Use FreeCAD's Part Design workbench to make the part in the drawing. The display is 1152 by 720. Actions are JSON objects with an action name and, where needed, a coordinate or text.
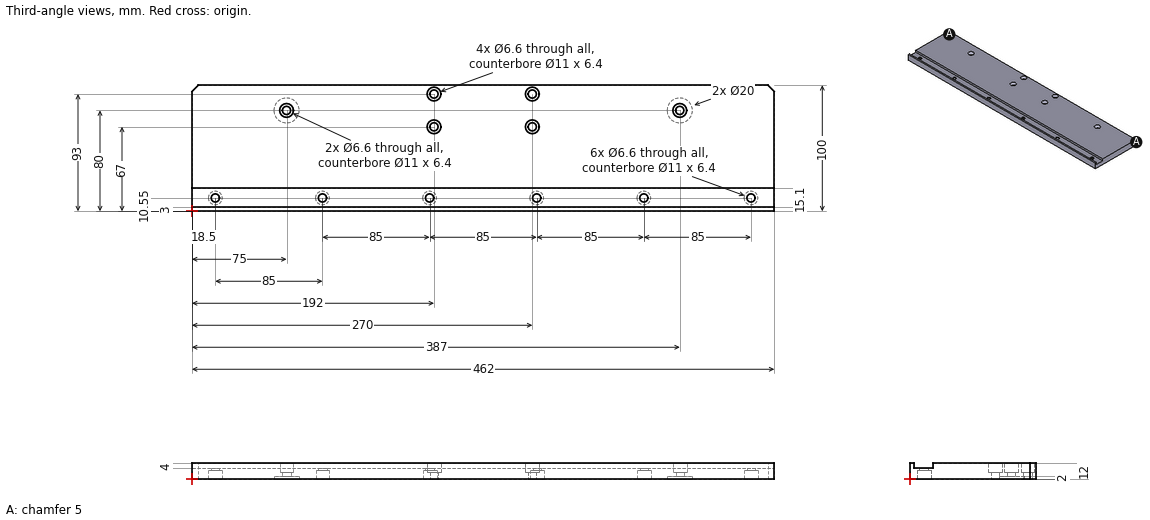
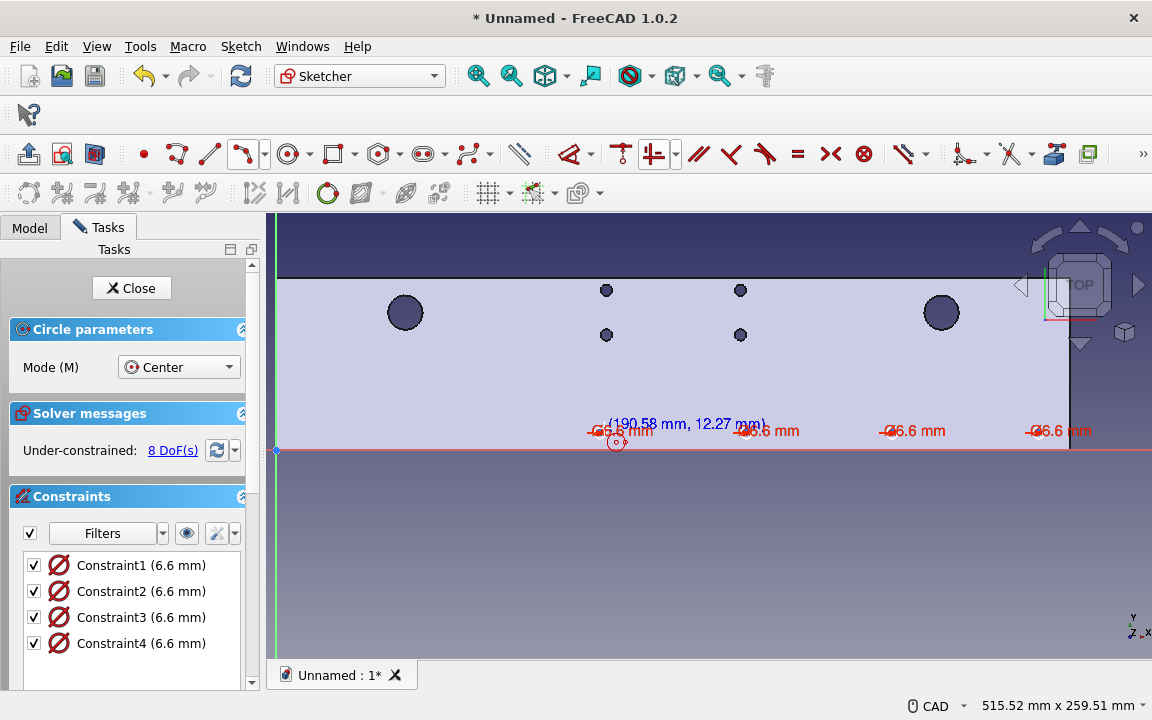
{"action": "scroll", "coordinate": [454, 432], "scroll_direction": "up", "scroll_amount": 7}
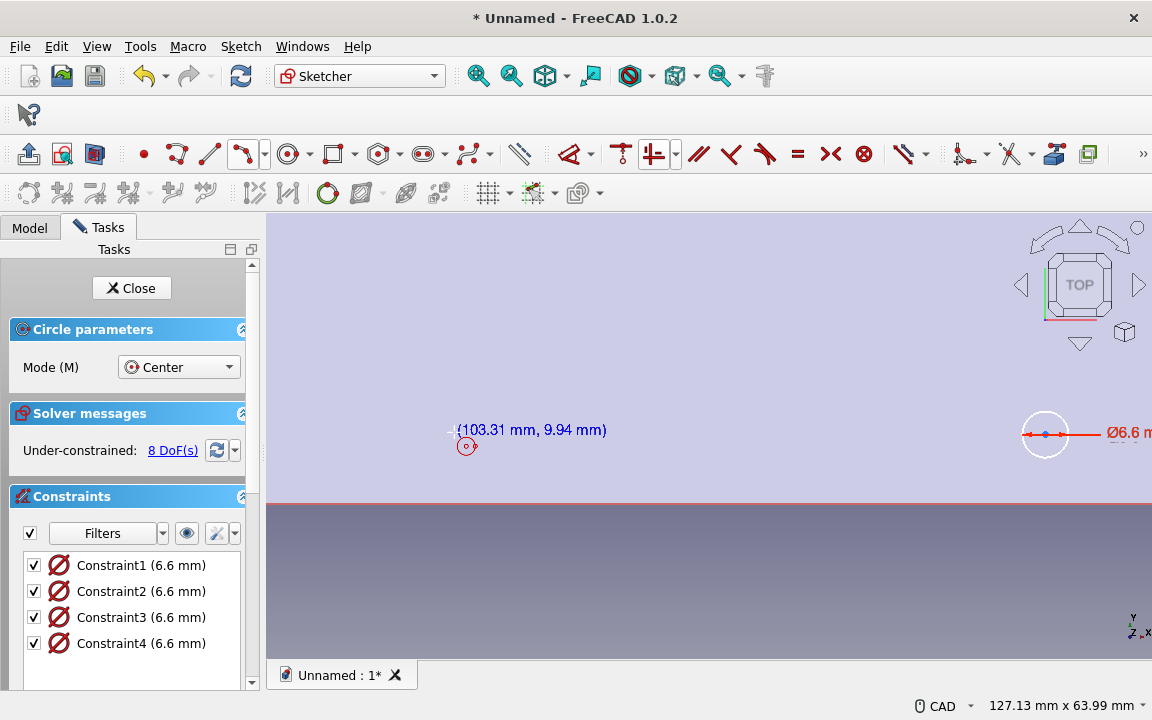
{"action": "scroll", "coordinate": [512, 432], "scroll_direction": "down", "scroll_amount": 9}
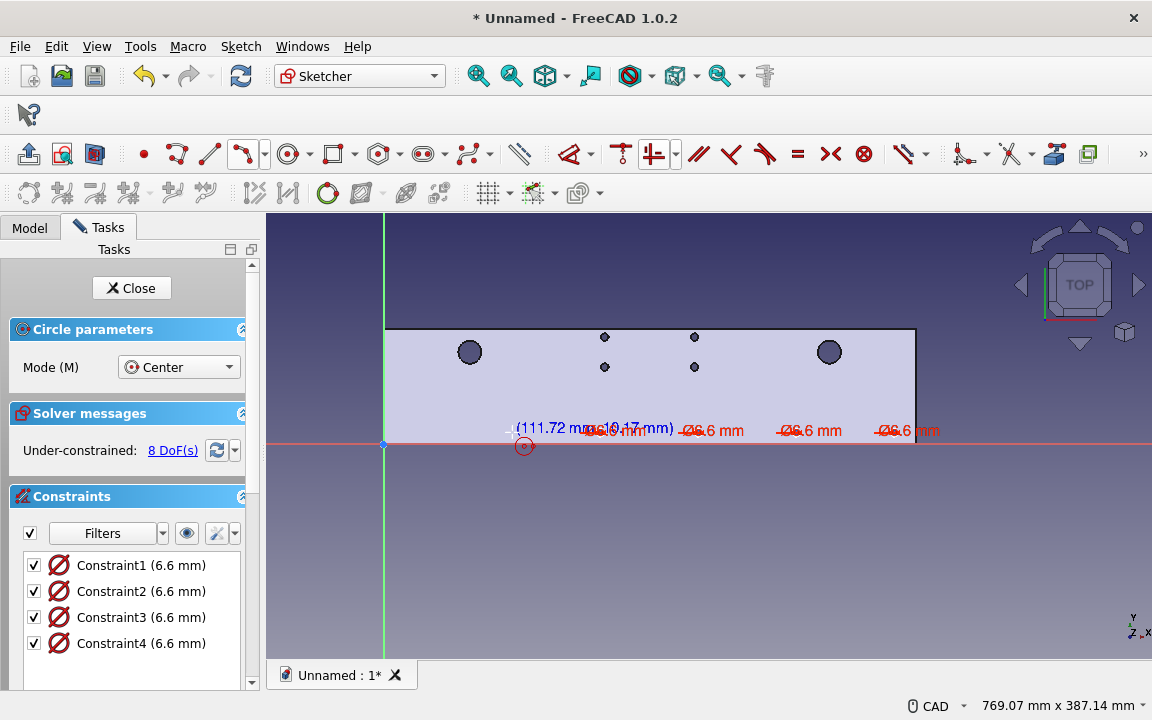
{"action": "scroll", "coordinate": [503, 432], "scroll_direction": "up", "scroll_amount": 2}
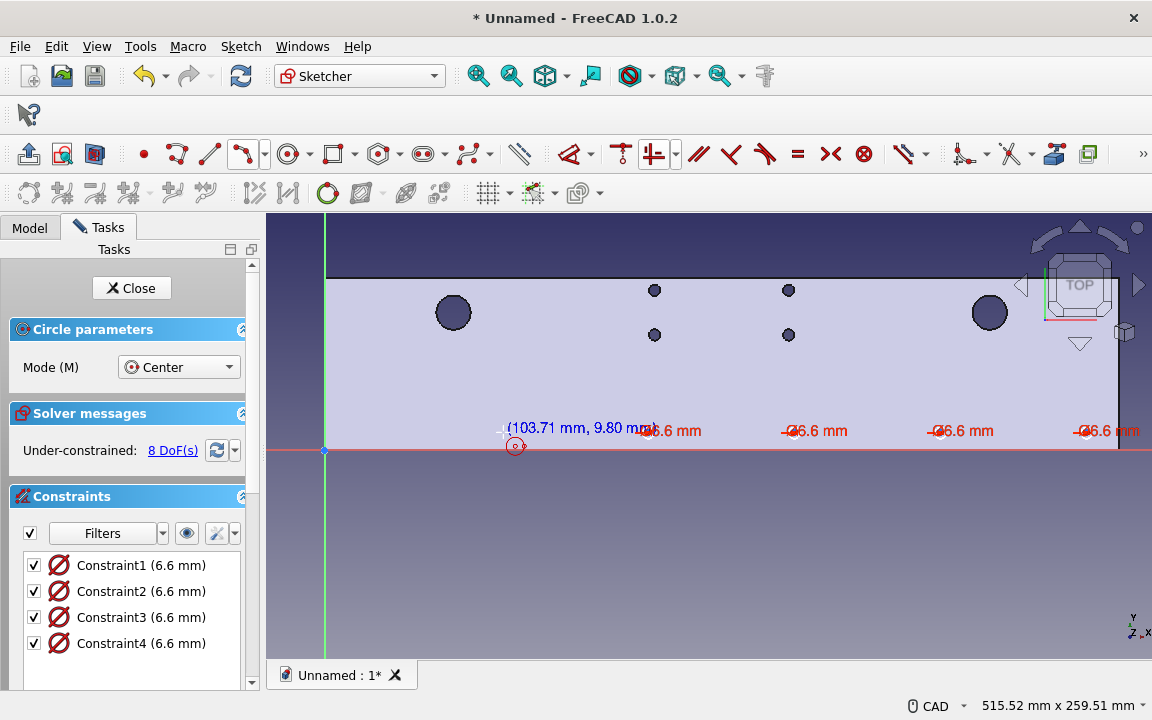
{"action": "left_click", "coordinate": [503, 432]}
{"action": "mouse_move", "coordinate": [507, 428]}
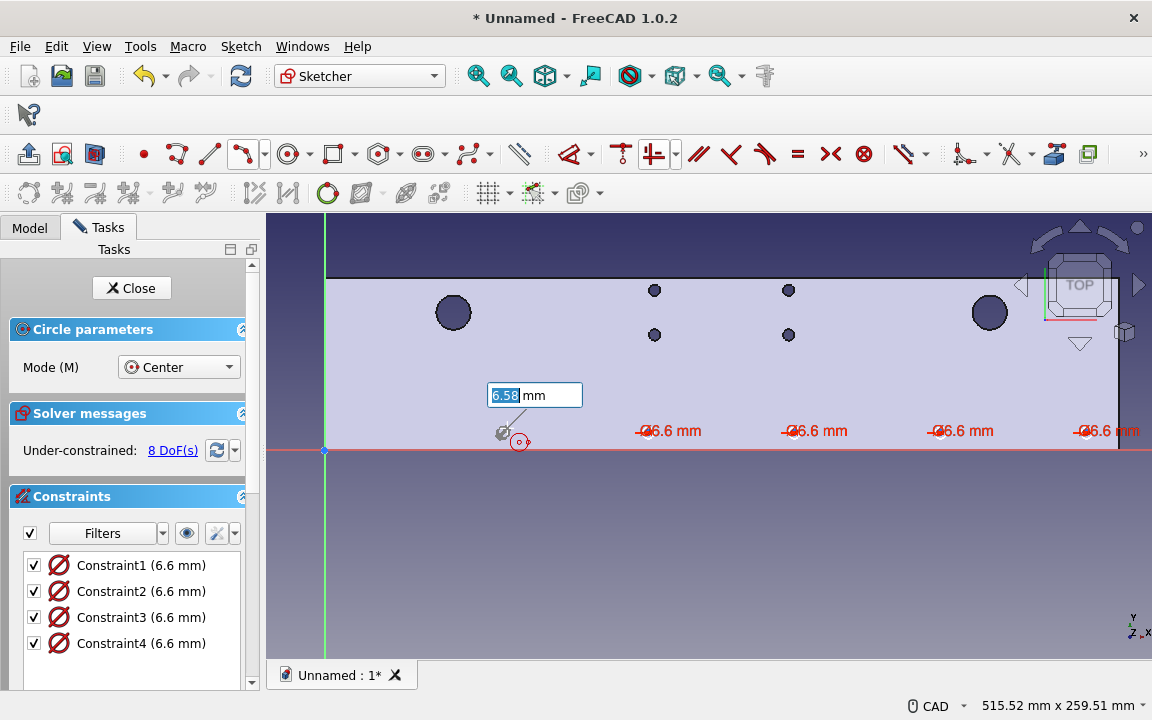
{"action": "type", "text": "6.6"}
{"action": "key", "text": "Return"}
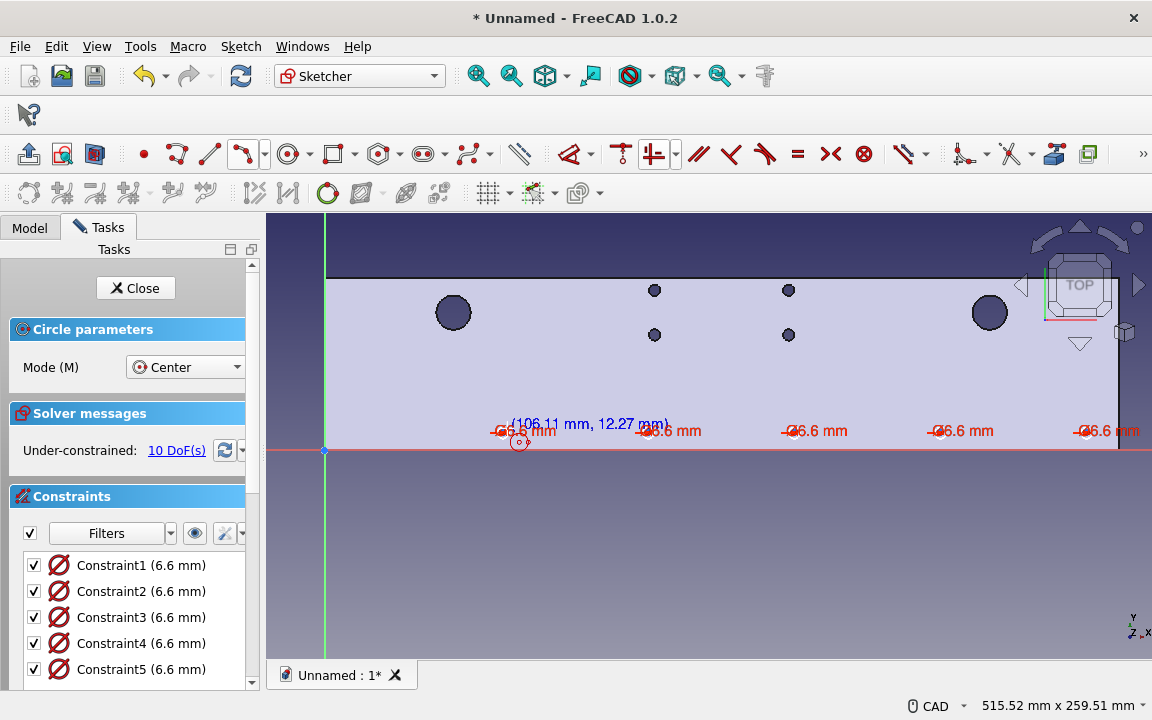
{"action": "scroll", "coordinate": [356, 432], "scroll_direction": "up", "scroll_amount": 7}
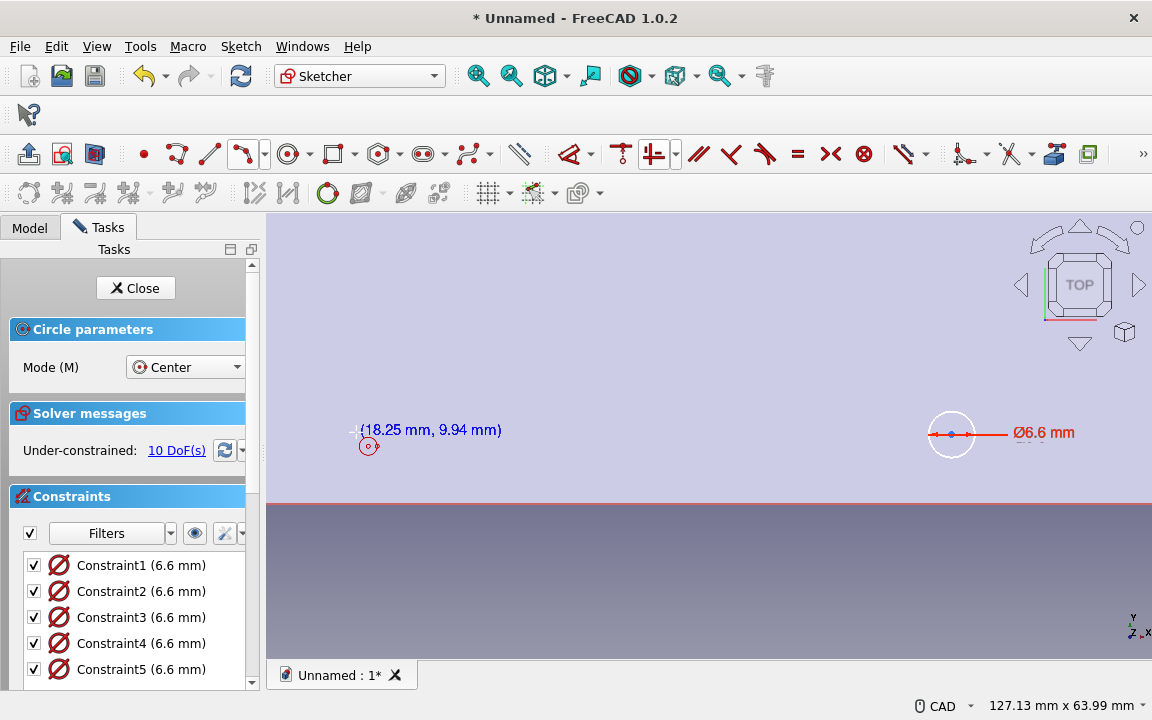
{"action": "scroll", "coordinate": [414, 432], "scroll_direction": "down", "scroll_amount": 9}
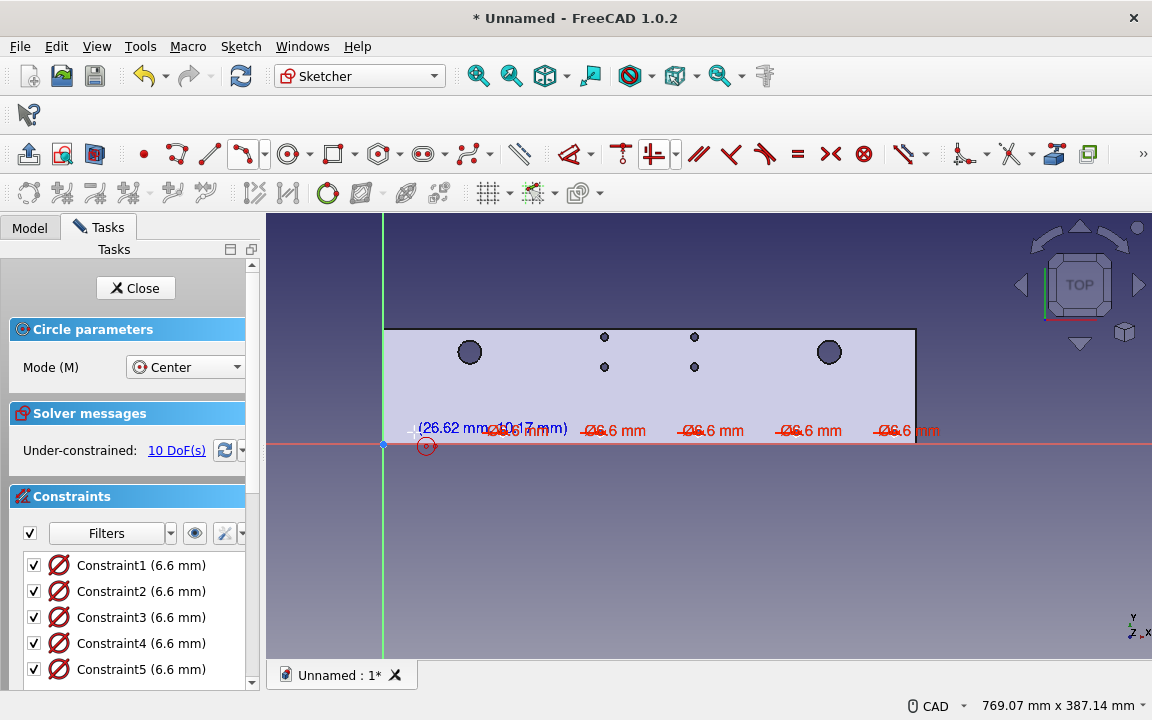
{"action": "scroll", "coordinate": [405, 432], "scroll_direction": "up", "scroll_amount": 2}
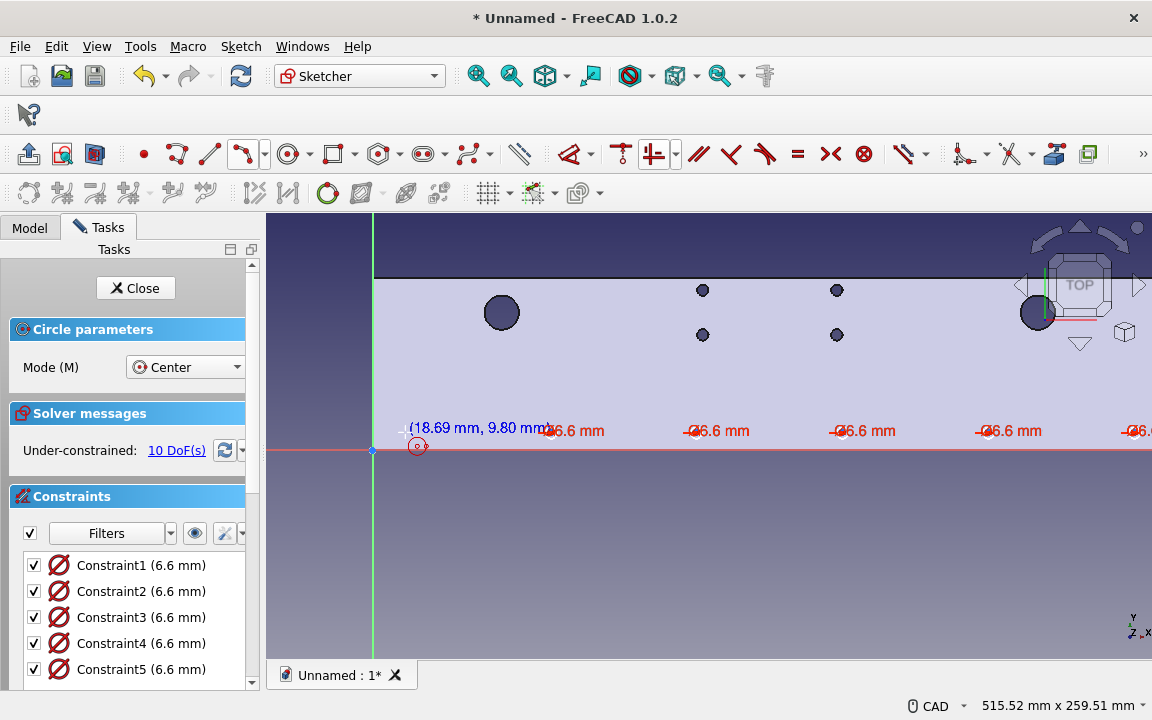
{"action": "left_click", "coordinate": [405, 432]}
{"action": "mouse_move", "coordinate": [409, 428]}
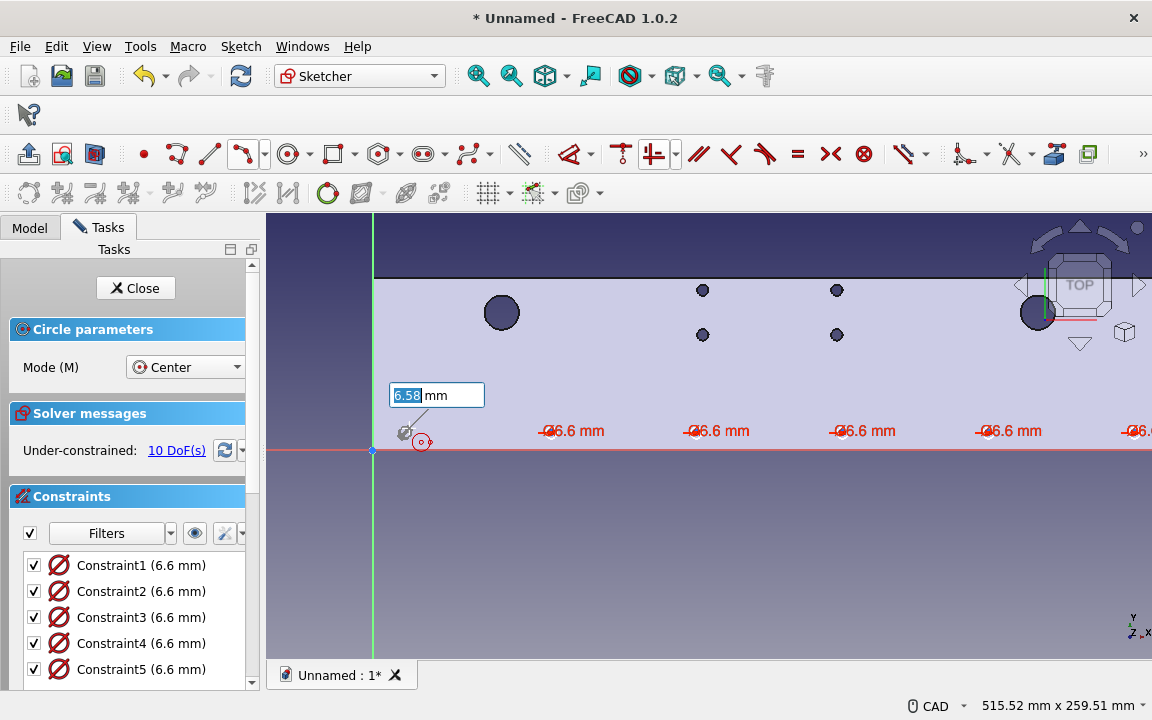
{"action": "type", "text": "6.6"}
{"action": "key", "text": "Return"}
{"action": "key", "text": "Escape"}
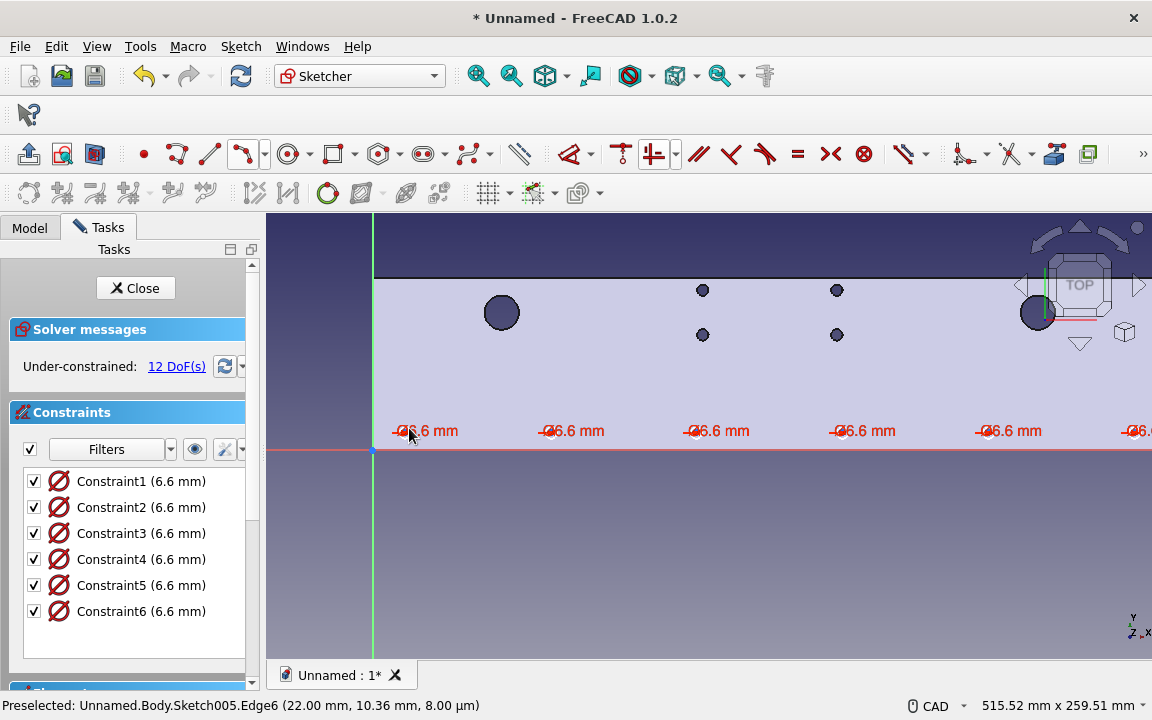
{"action": "scroll", "coordinate": [404, 432], "scroll_direction": "down", "scroll_amount": 2}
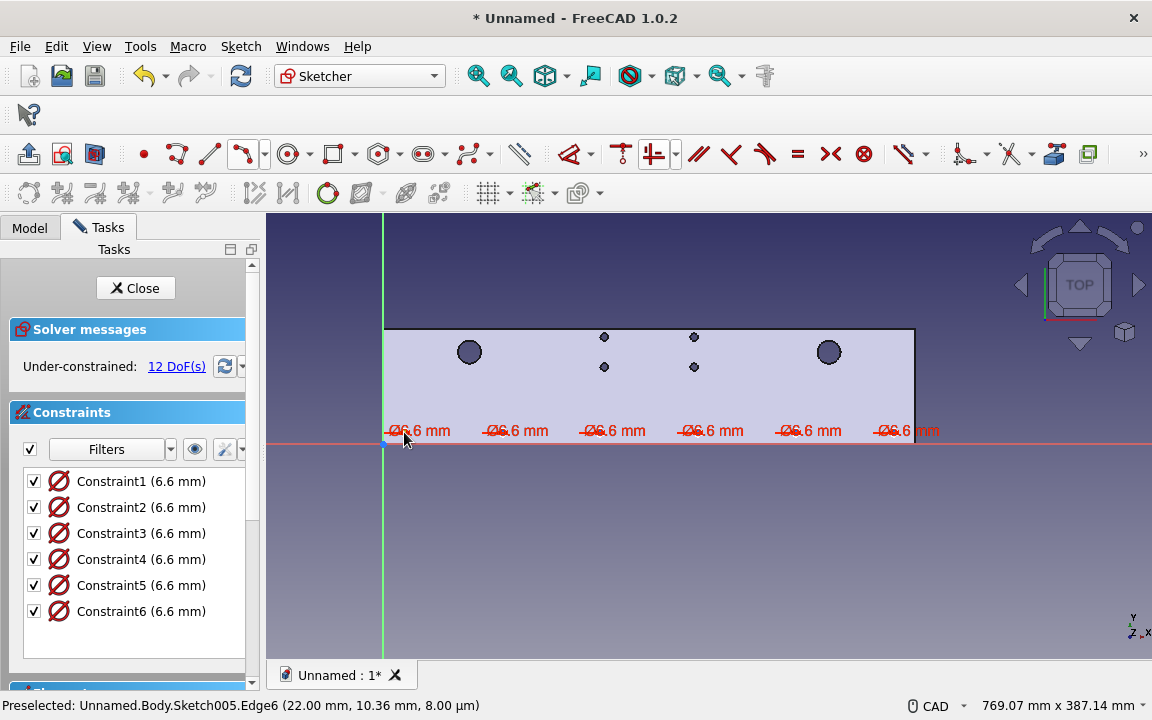
{"action": "left_click", "coordinate": [894, 433]}